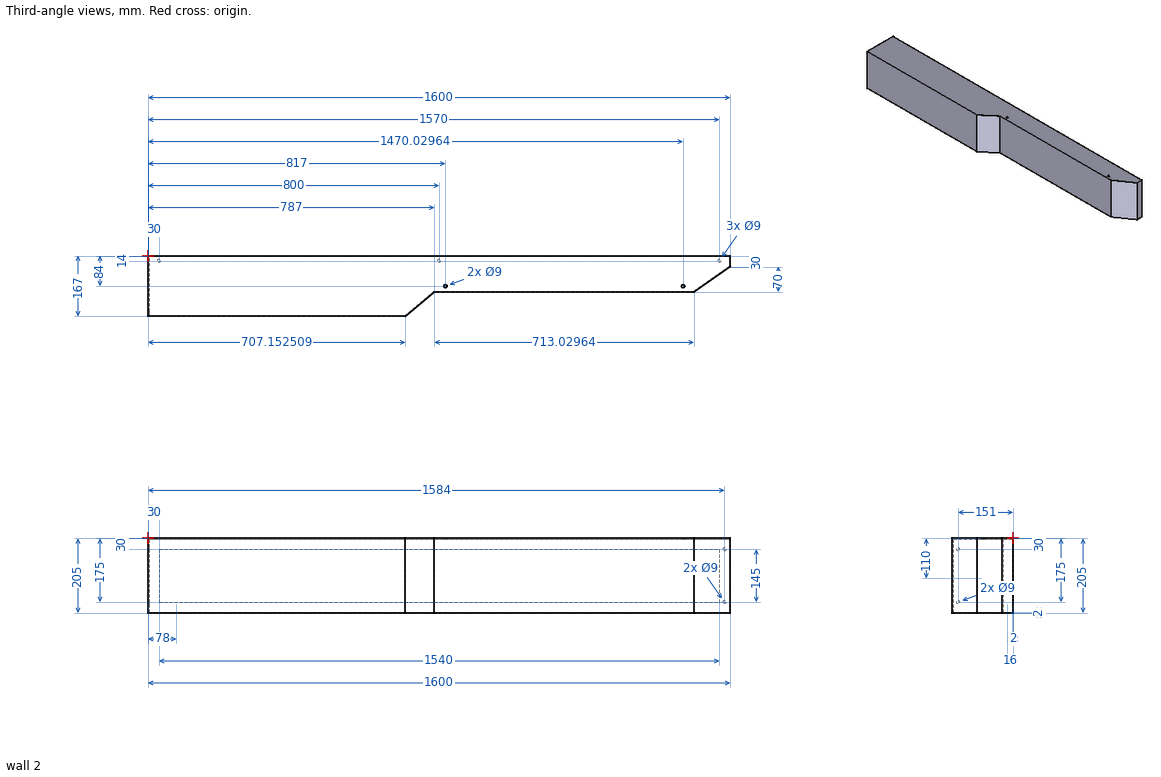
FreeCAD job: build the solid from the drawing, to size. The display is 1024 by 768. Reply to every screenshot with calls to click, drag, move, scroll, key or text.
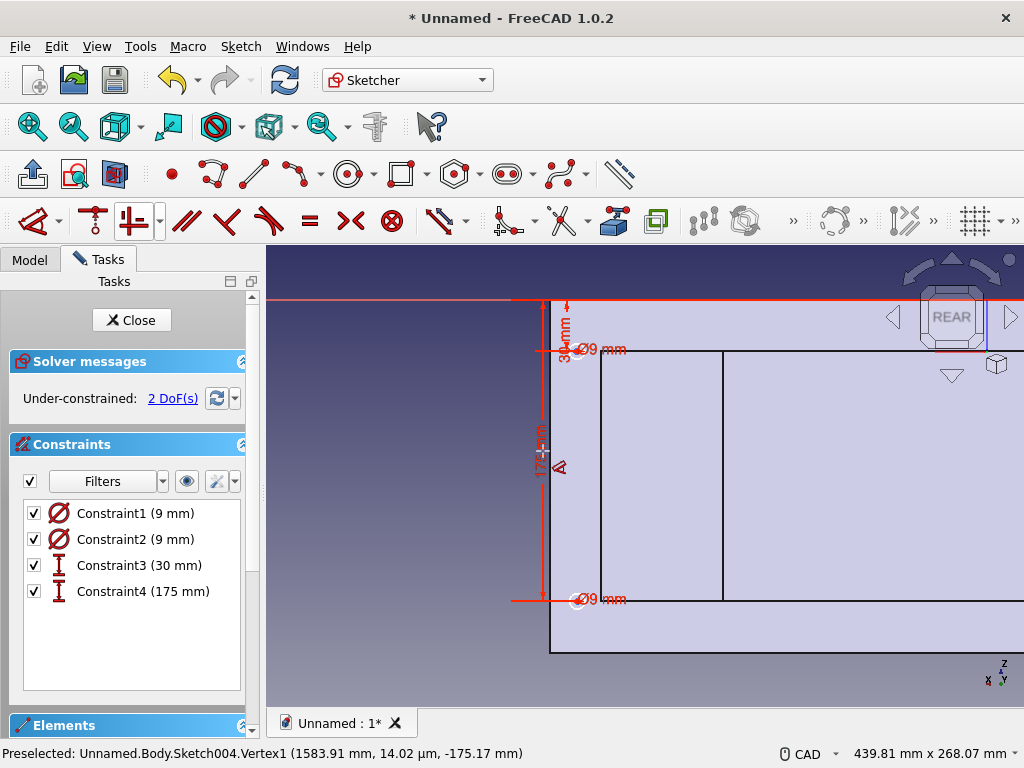
click(577, 601)
click(718, 635)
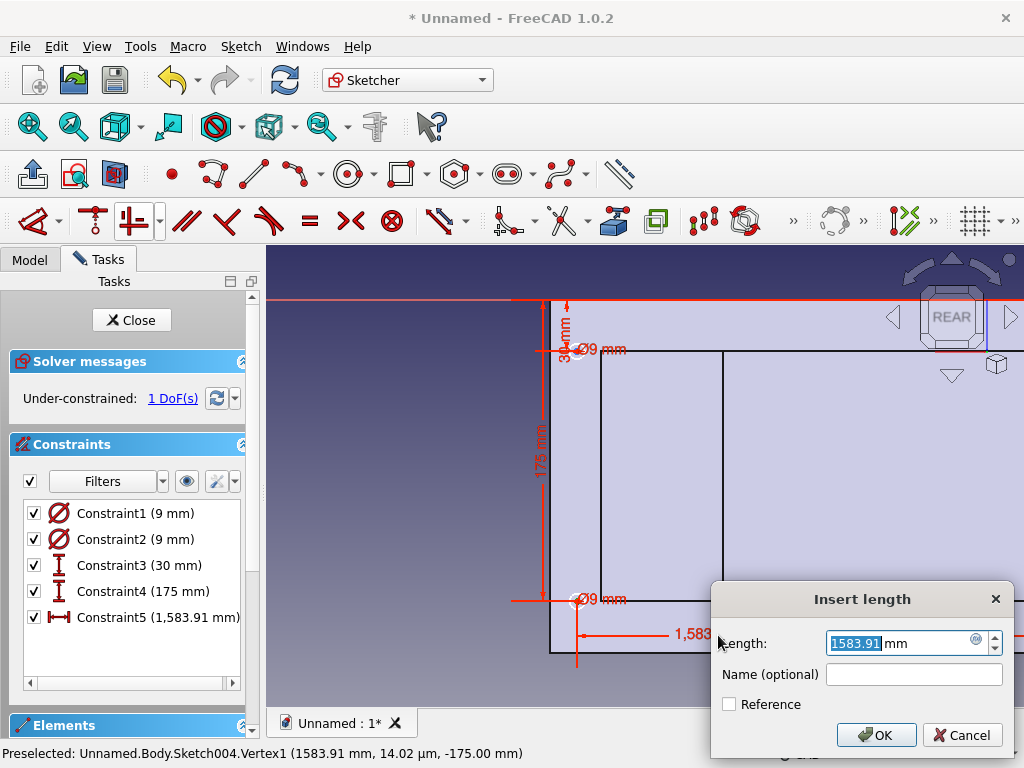
text(1584)
key(Return)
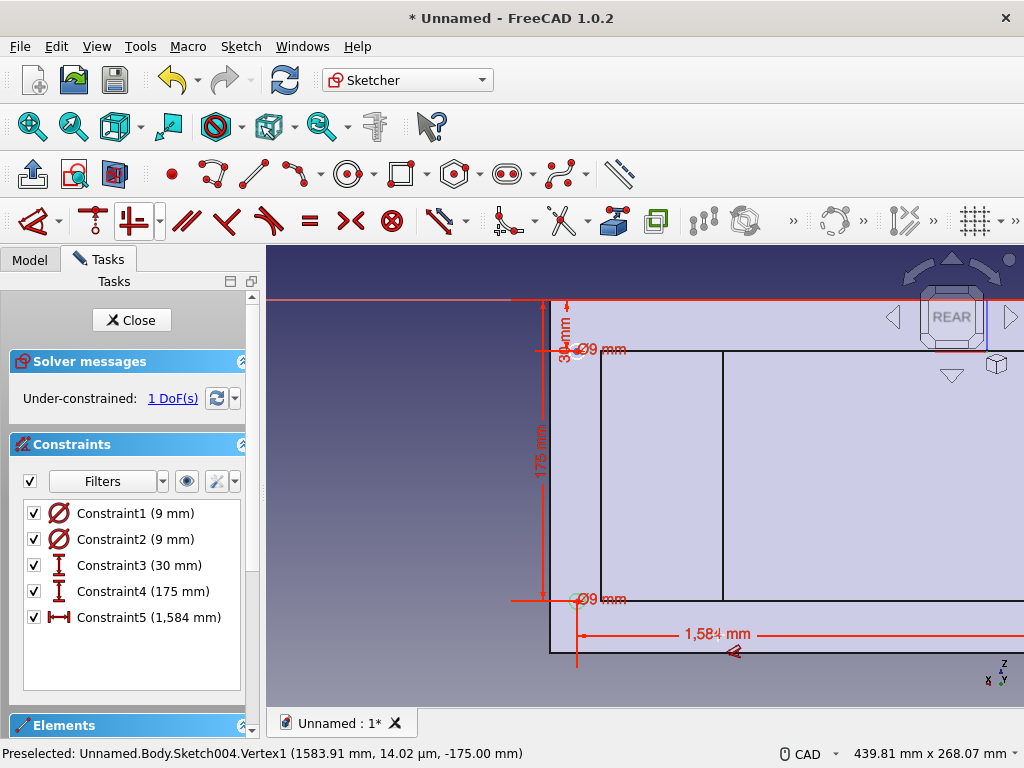
click(577, 351)
click(718, 385)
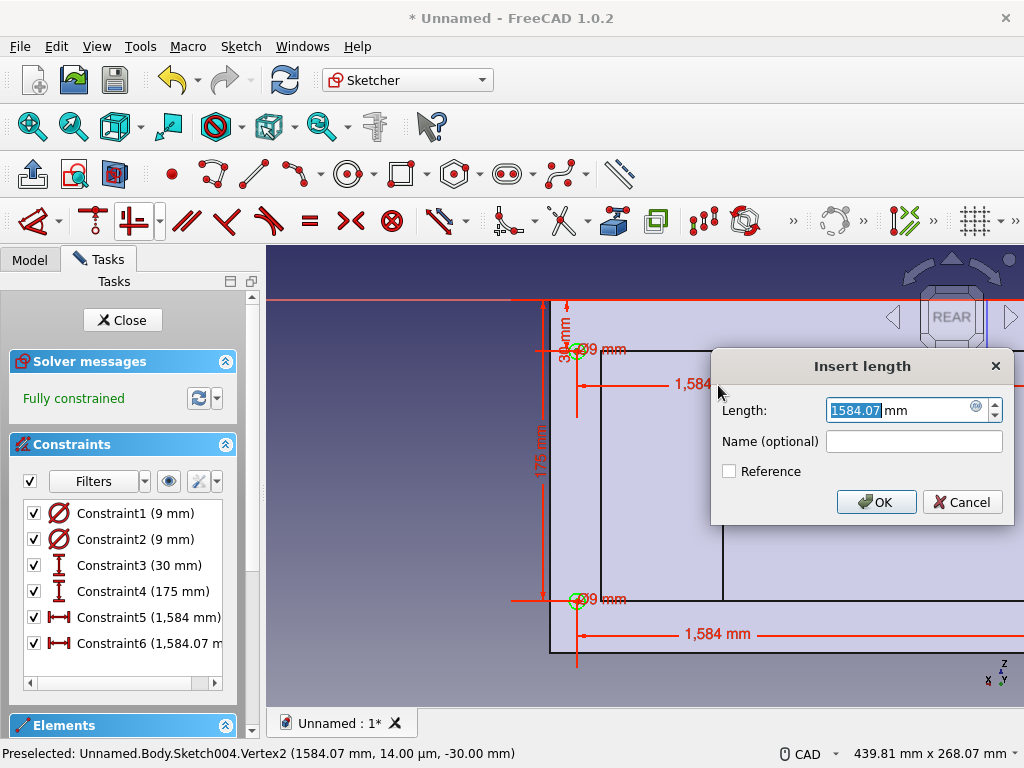
text(1584)
key(Return)
key(Escape)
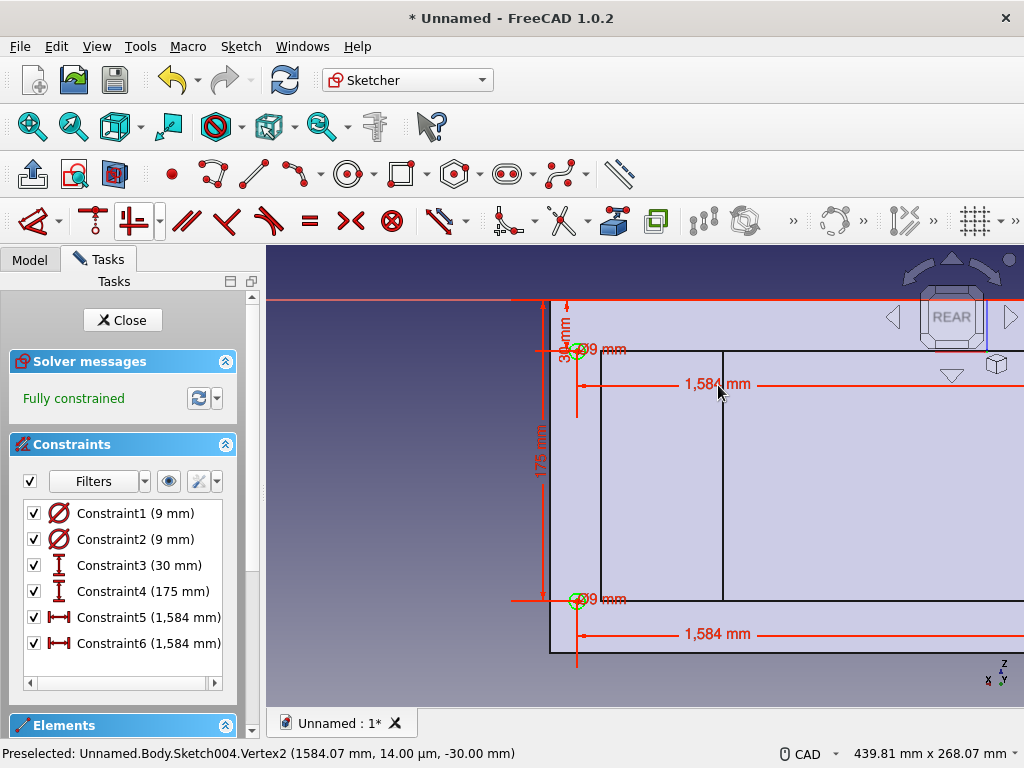
click(123, 320)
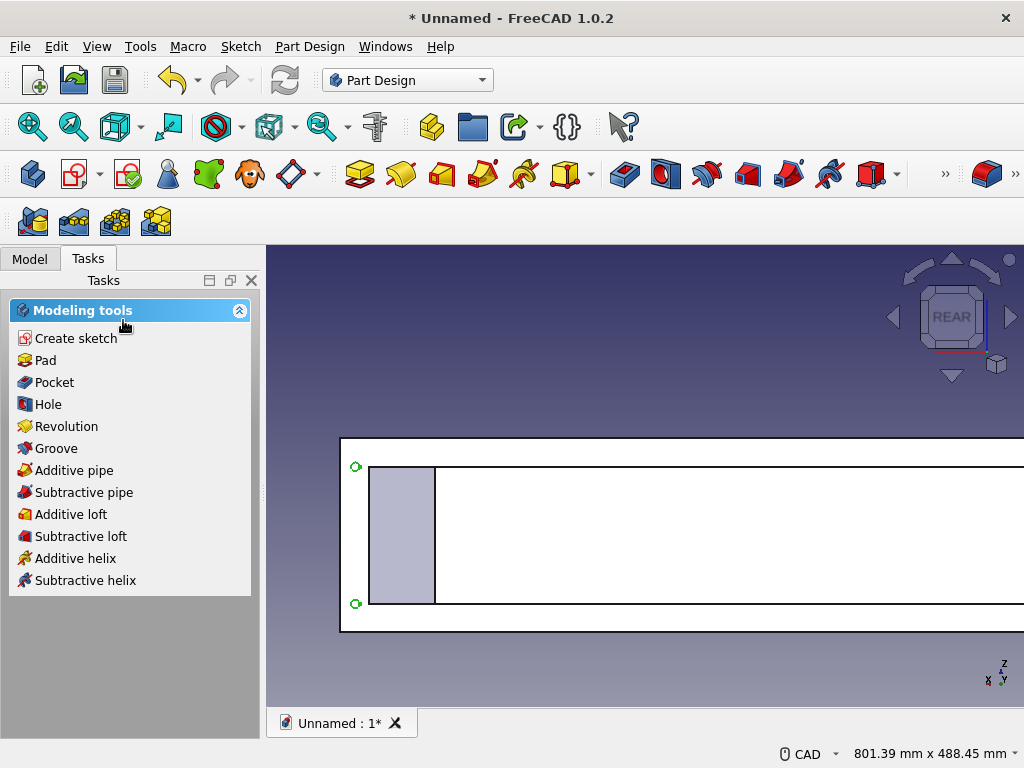
click(625, 174)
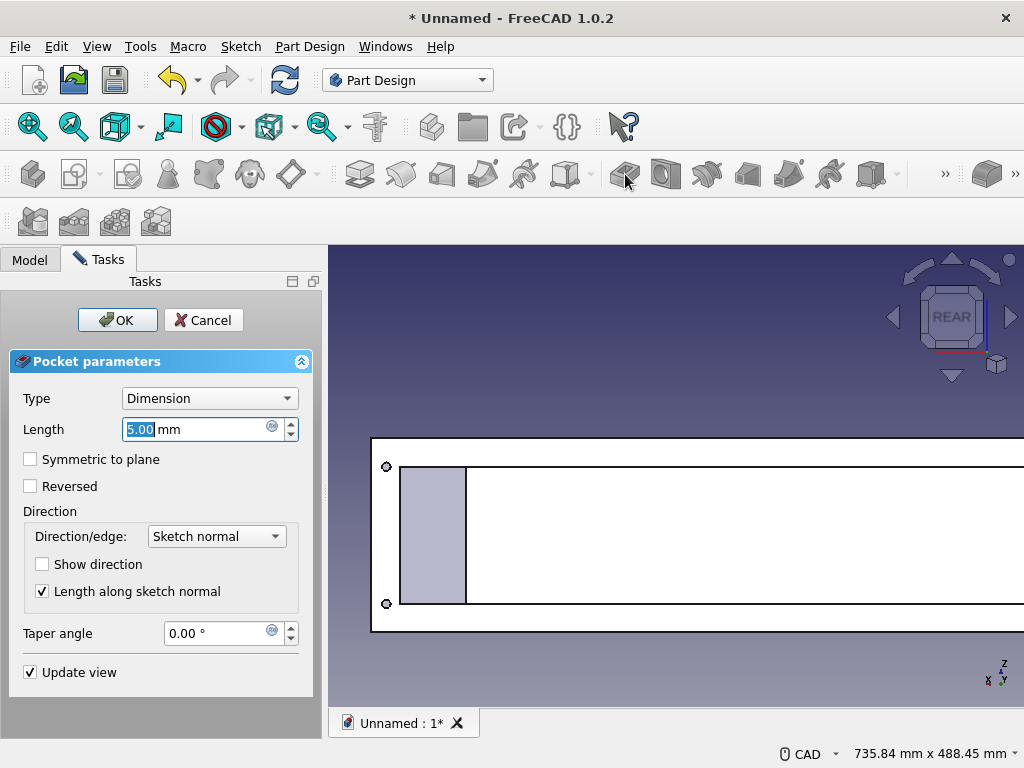
text(16)
key(Tab)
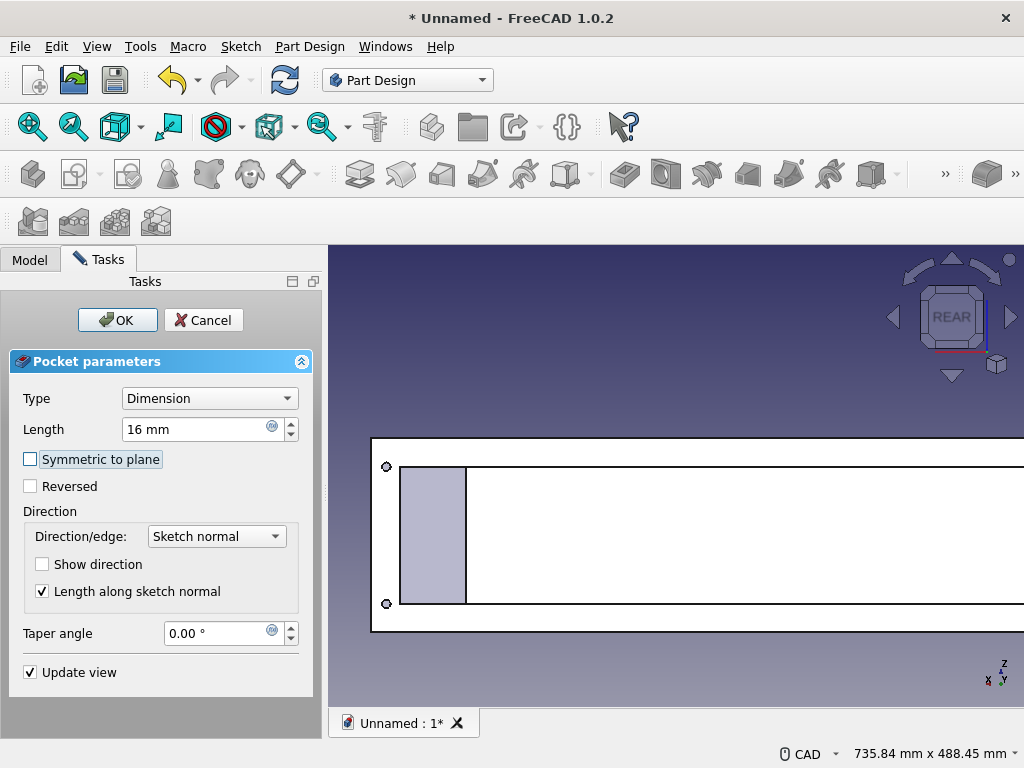
click(118, 320)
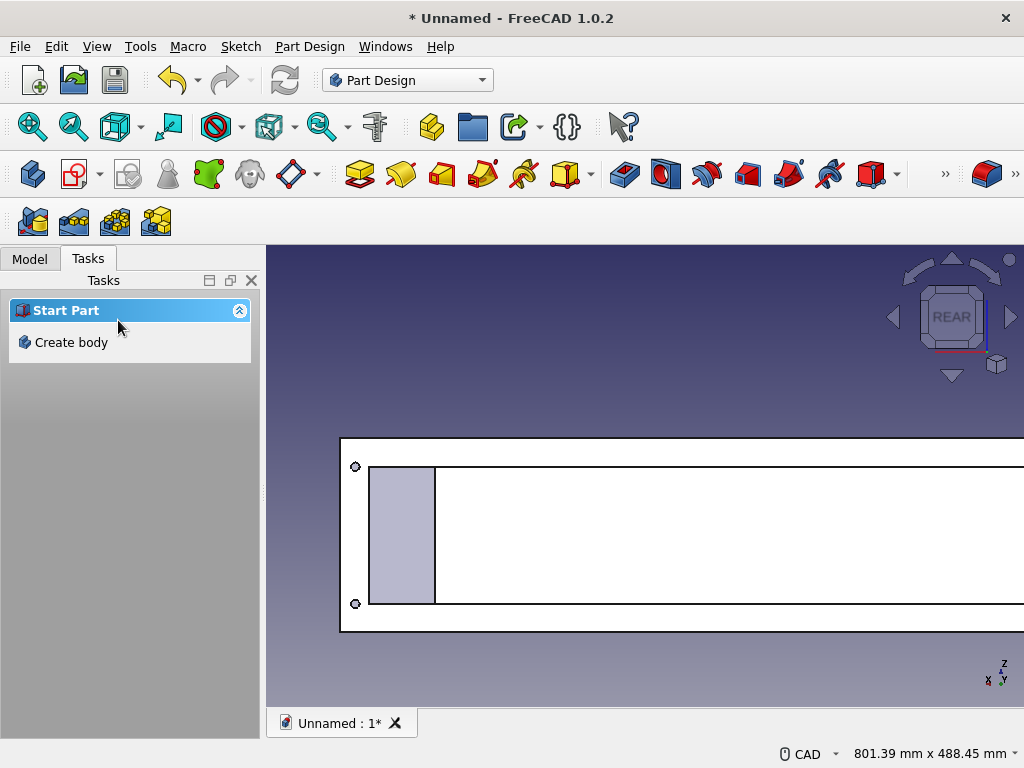
key(v)
key(f)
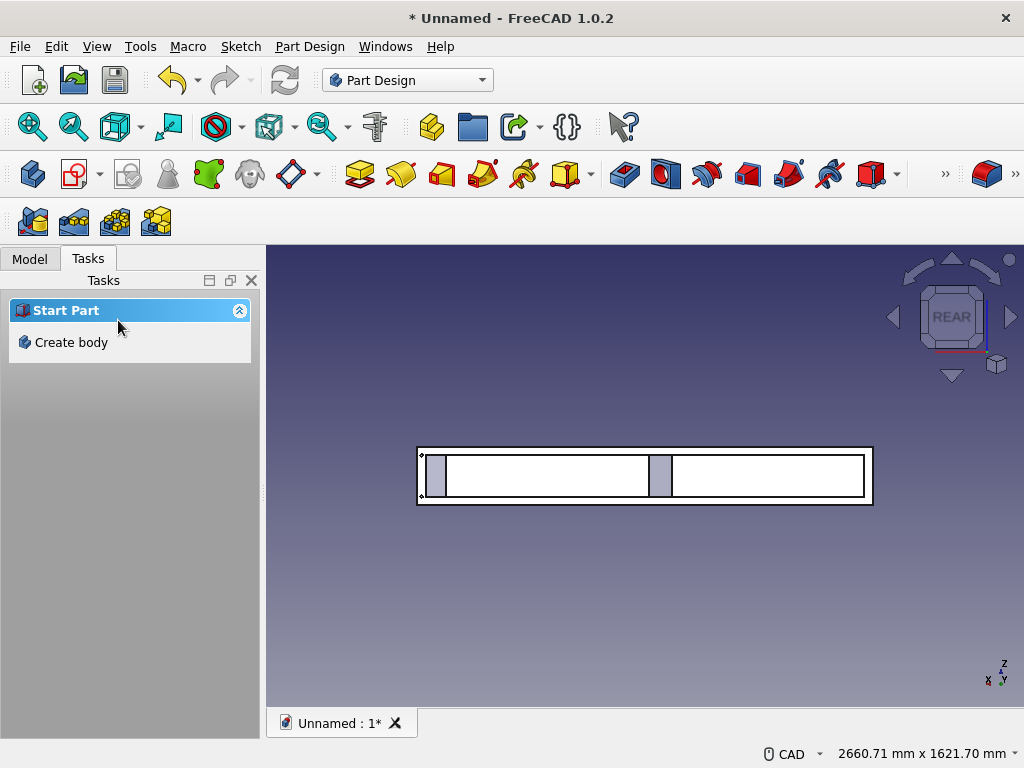
click(74, 174)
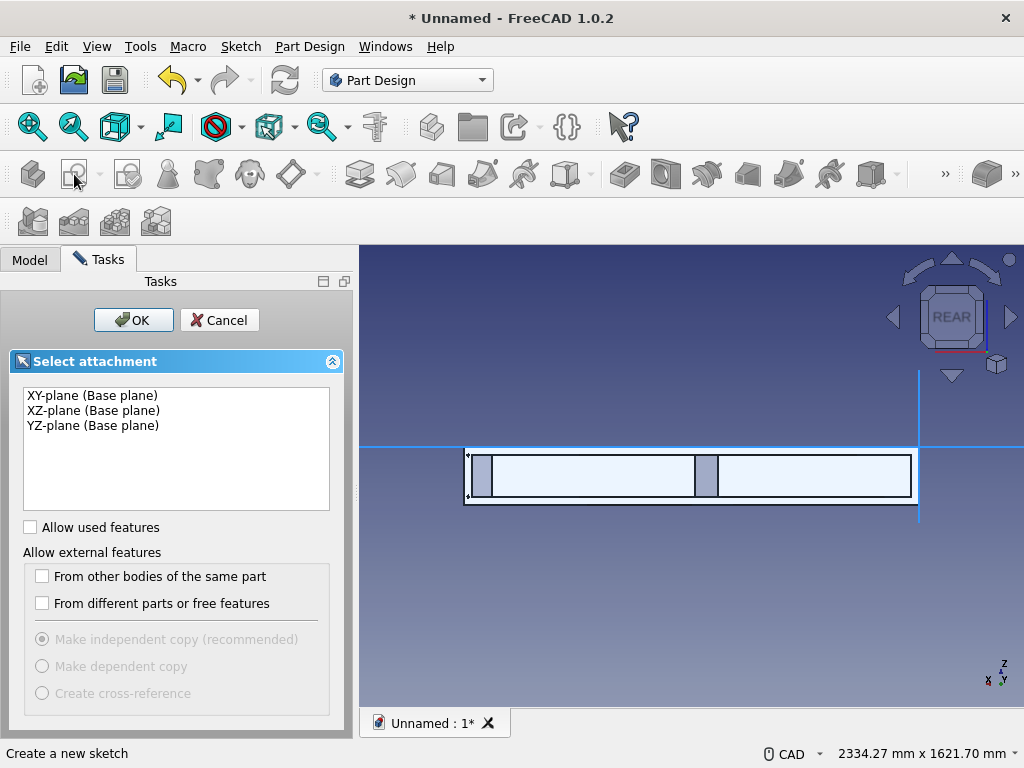
click(84, 396)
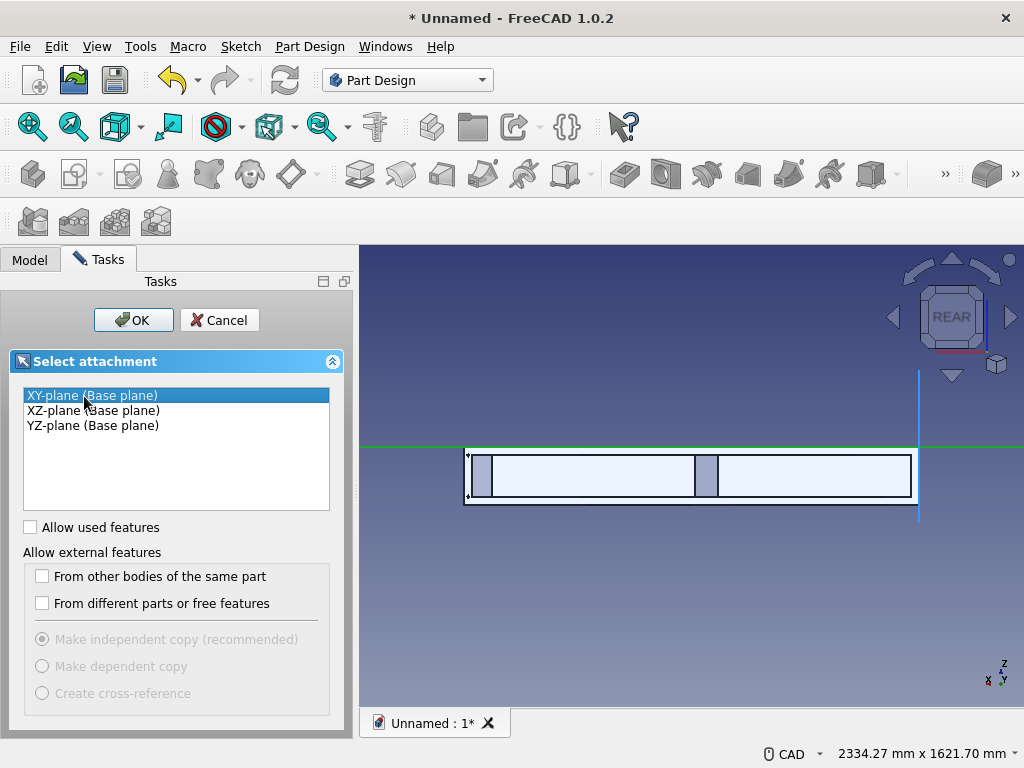
click(134, 320)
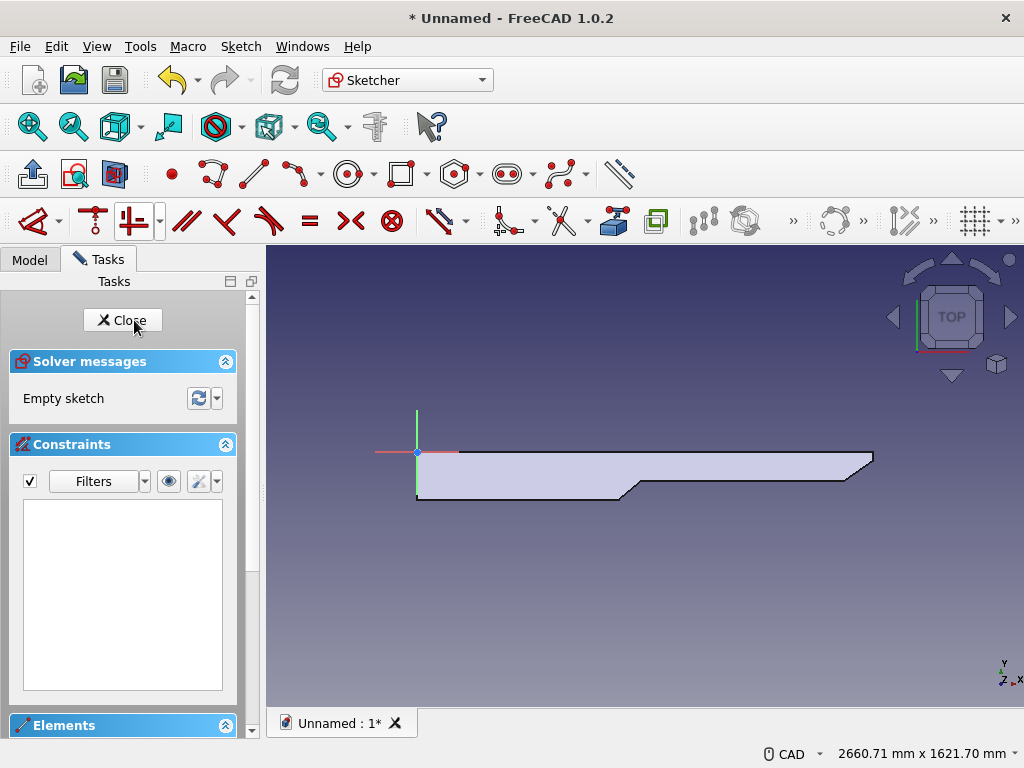
scroll(348, 527, down, 1)